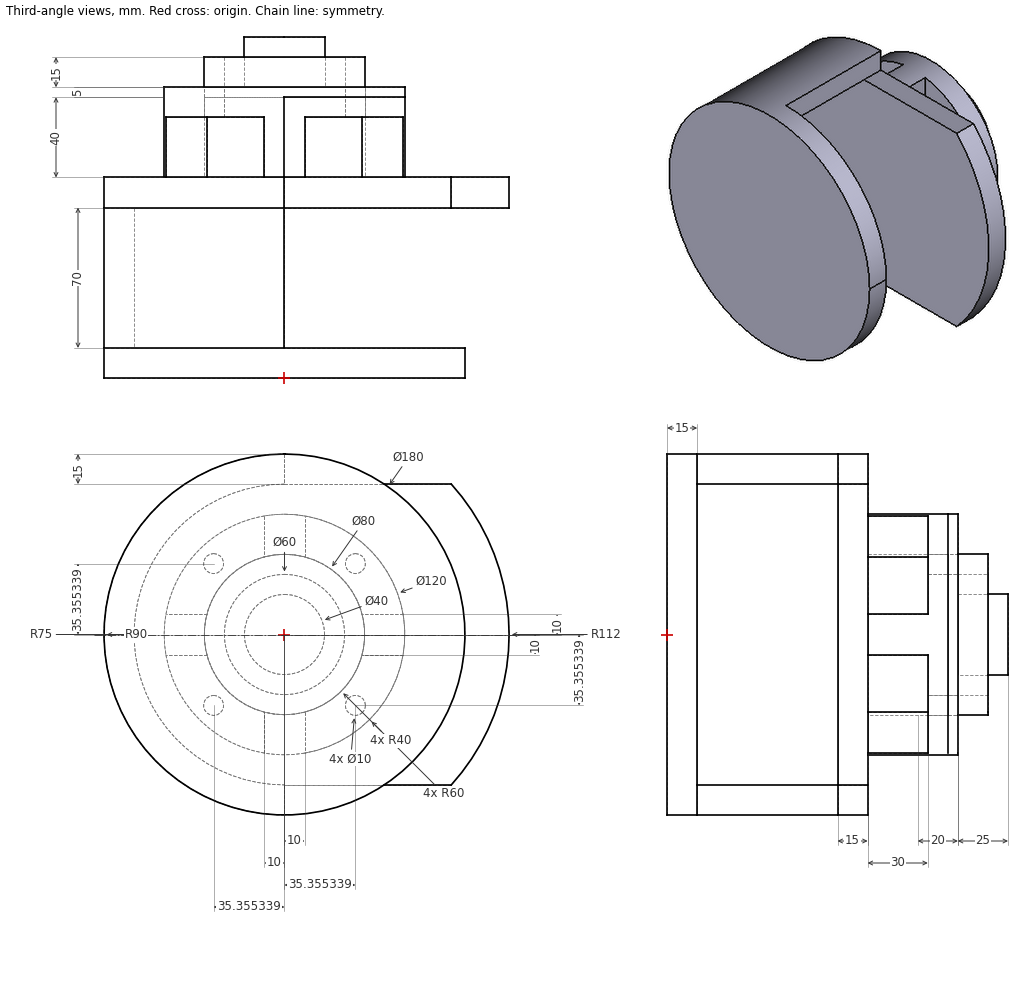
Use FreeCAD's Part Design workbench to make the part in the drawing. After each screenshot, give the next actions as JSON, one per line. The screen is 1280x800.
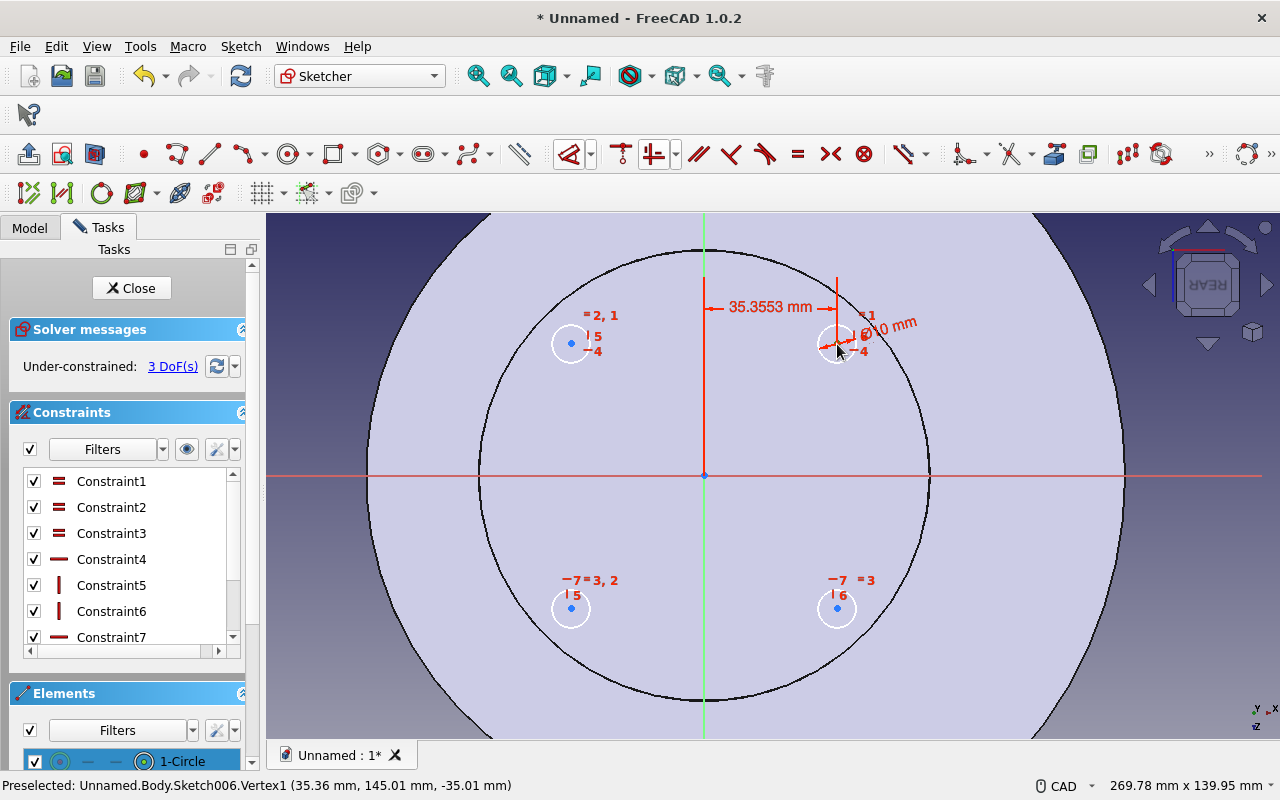
{"action": "left_click", "coordinate": [590, 154]}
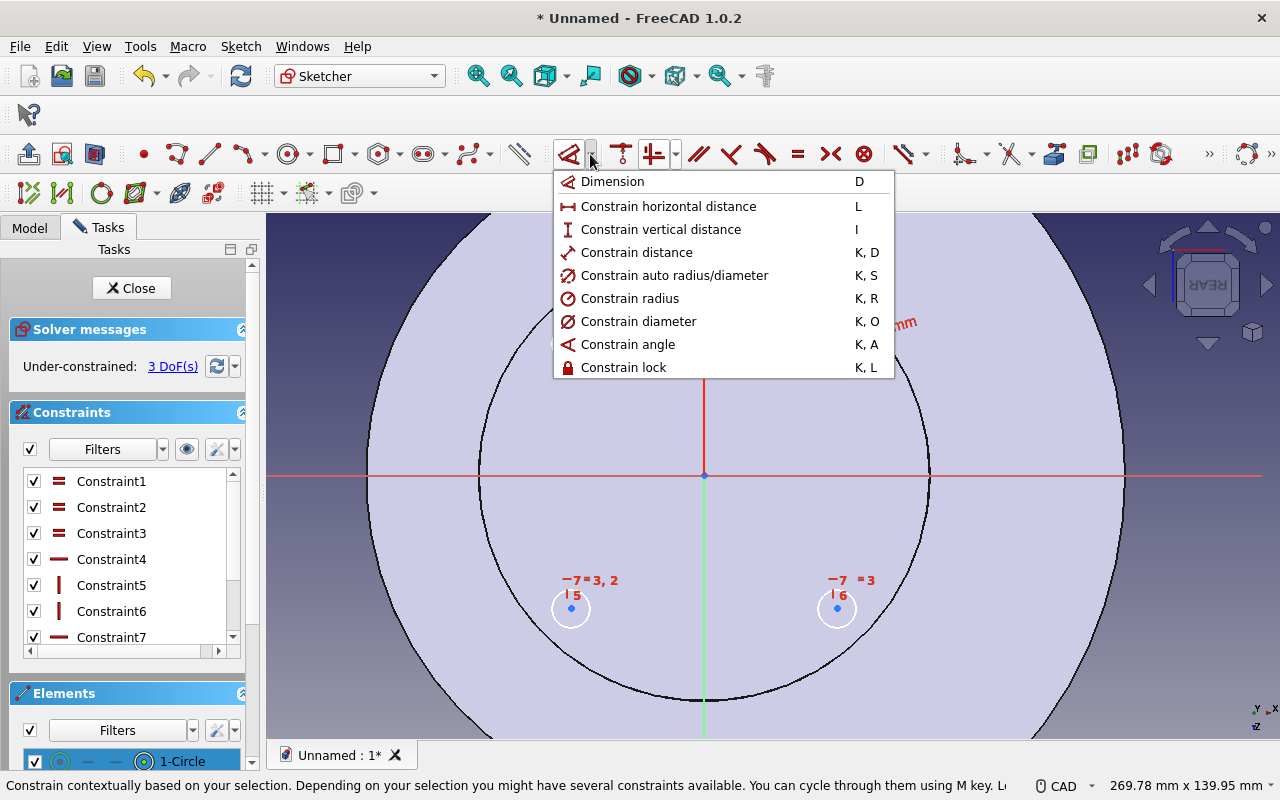
{"action": "left_click", "coordinate": [724, 230]}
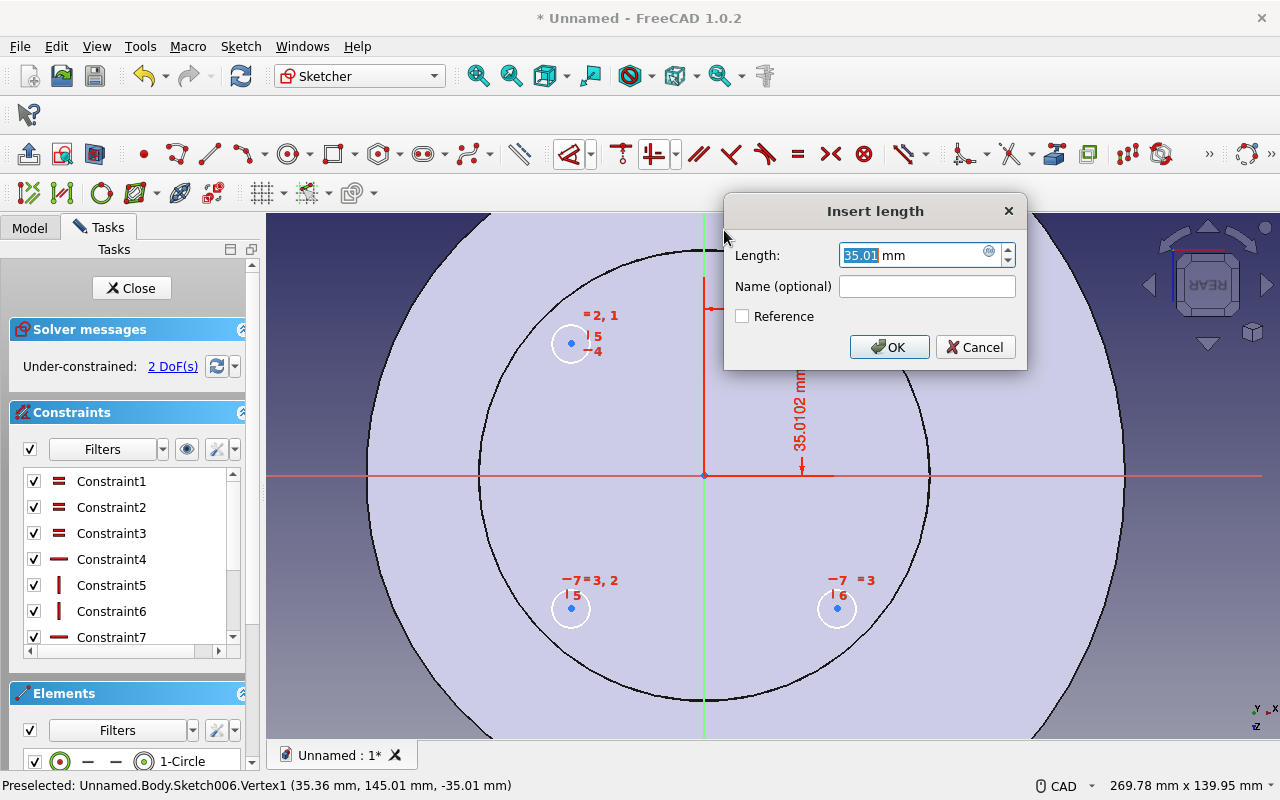
{"action": "type", "text": "35.355339"}
{"action": "key", "text": "Return"}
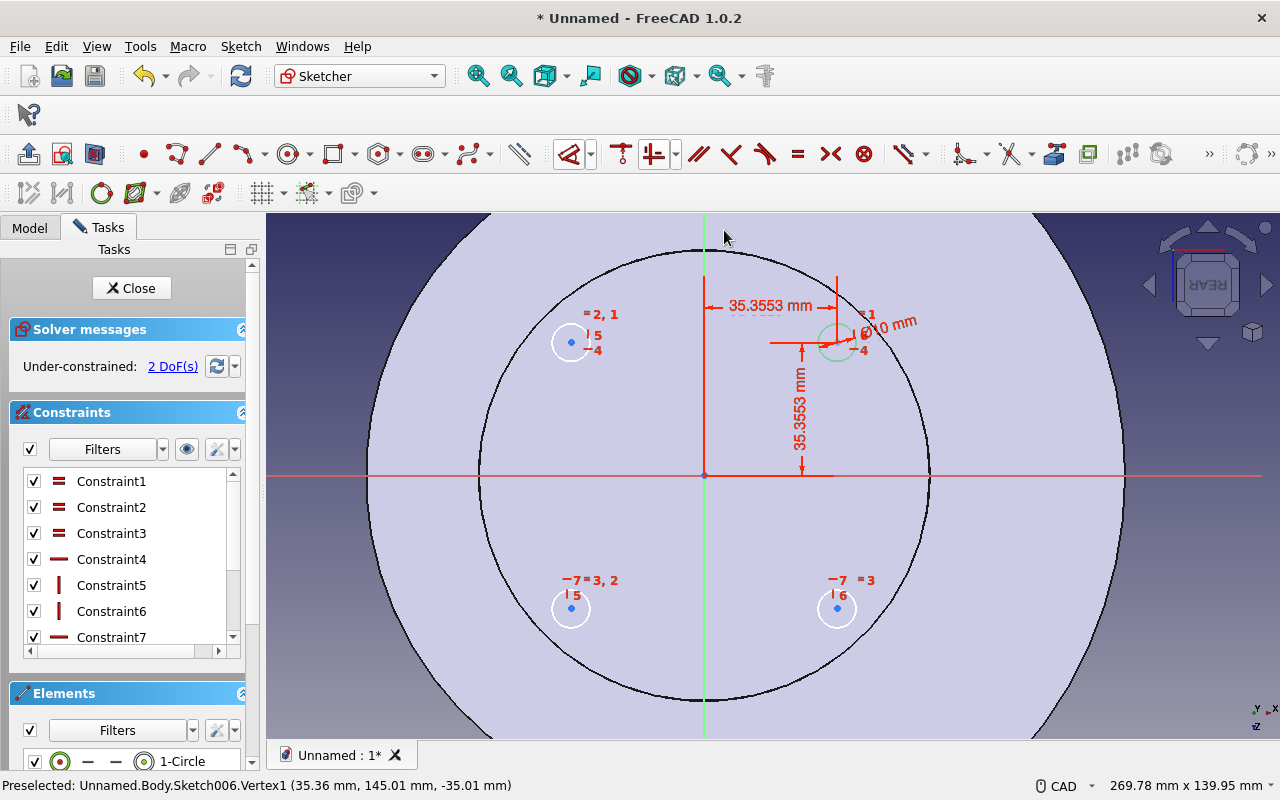
{"action": "left_click", "coordinate": [571, 343]}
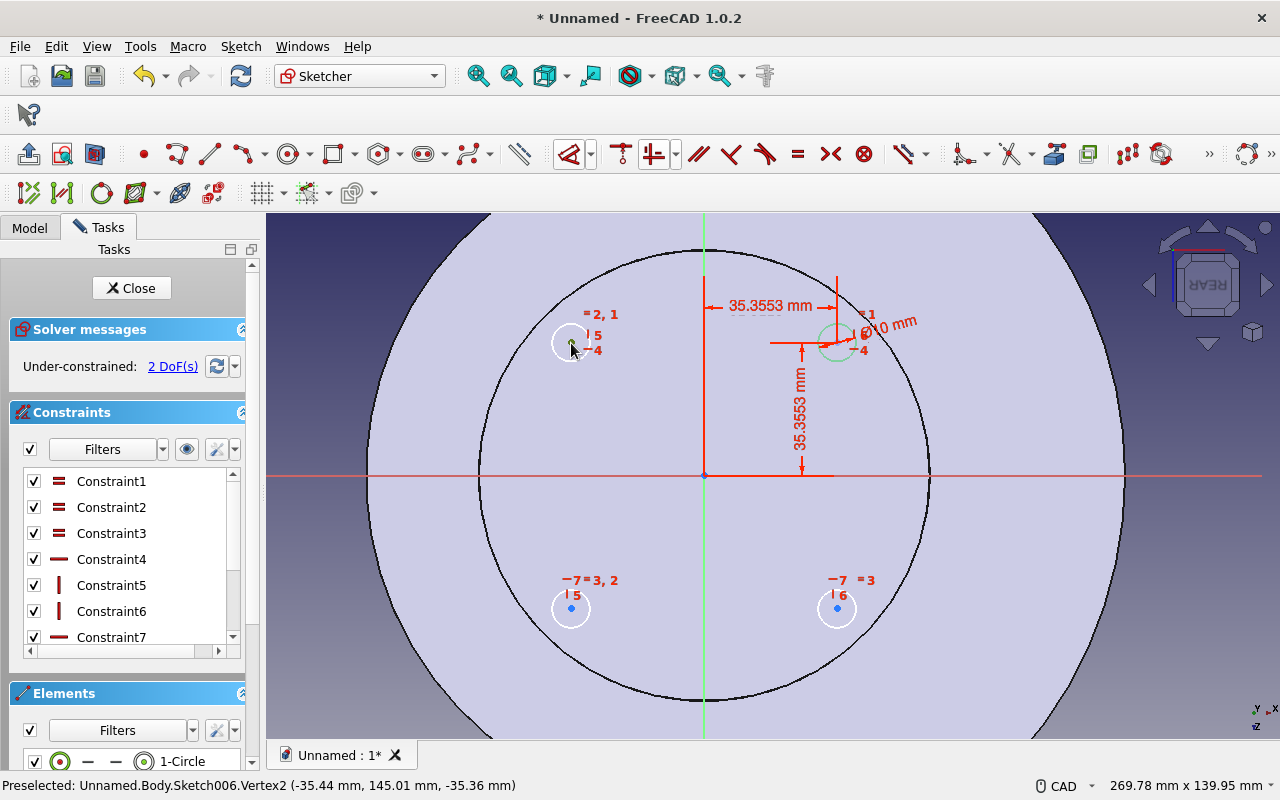
{"action": "key", "text": "l"}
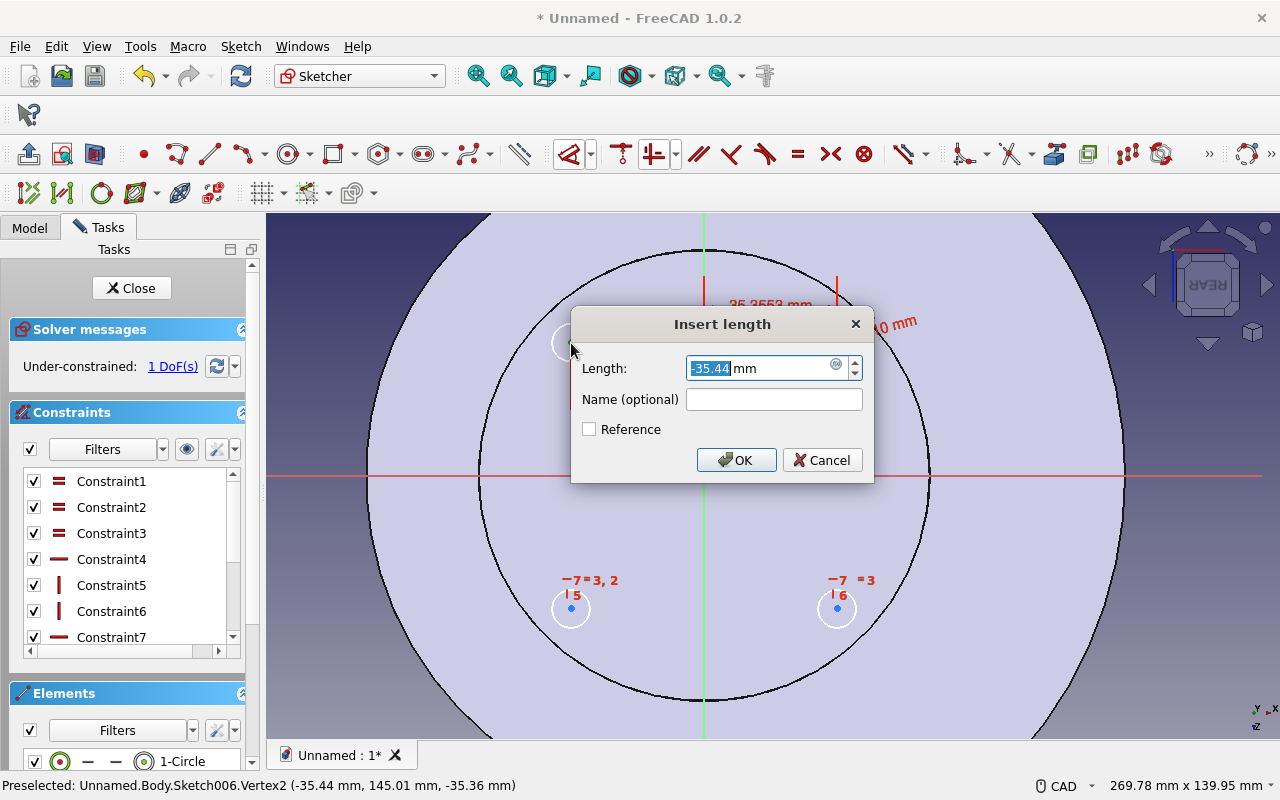
{"action": "type", "text": "-35.355339"}
{"action": "key", "text": "Return"}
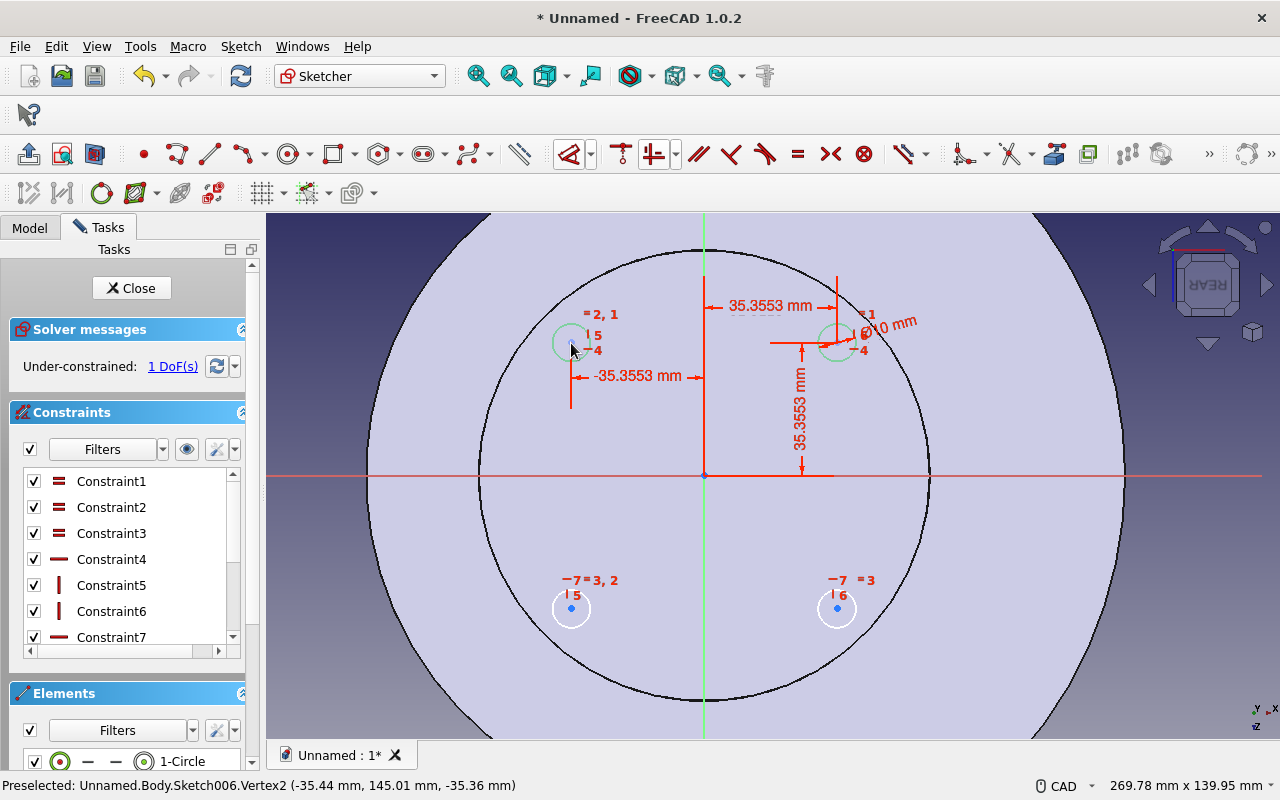
{"action": "left_click", "coordinate": [571, 609]}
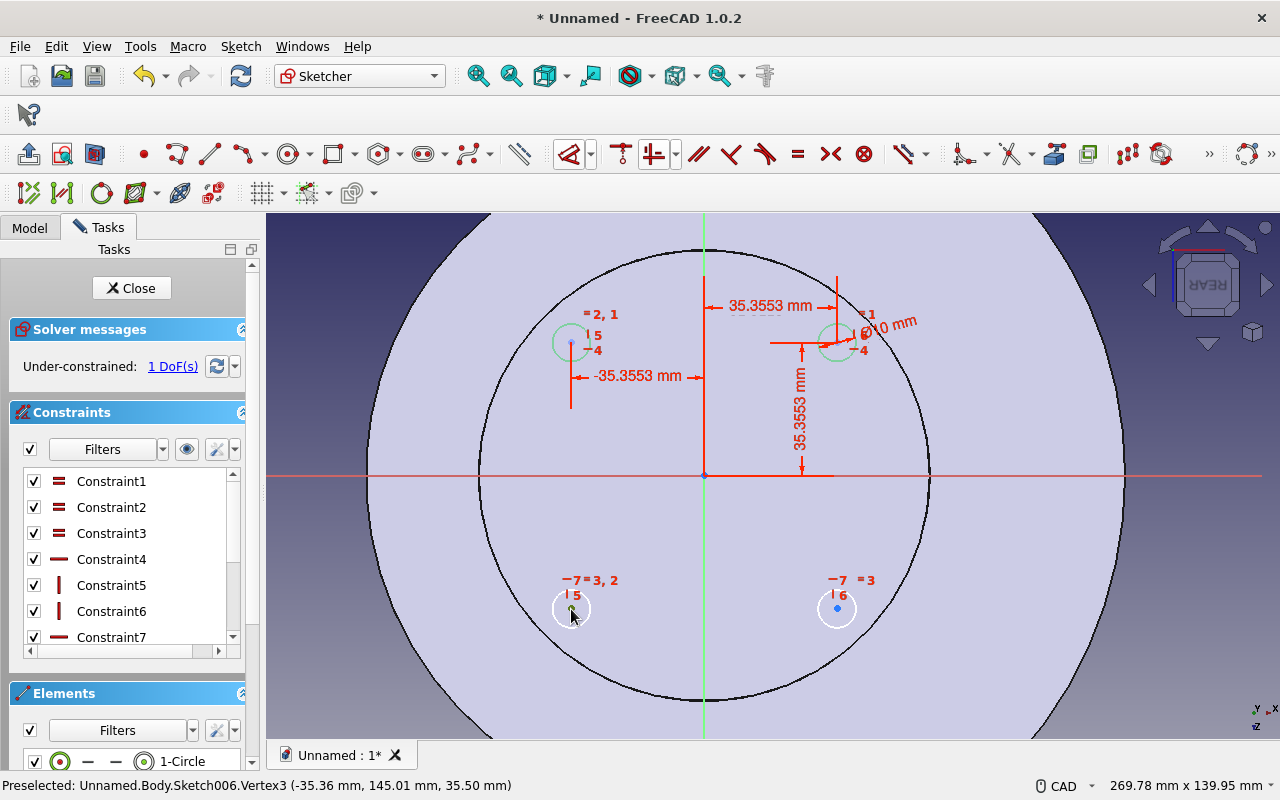
{"action": "key", "text": "i"}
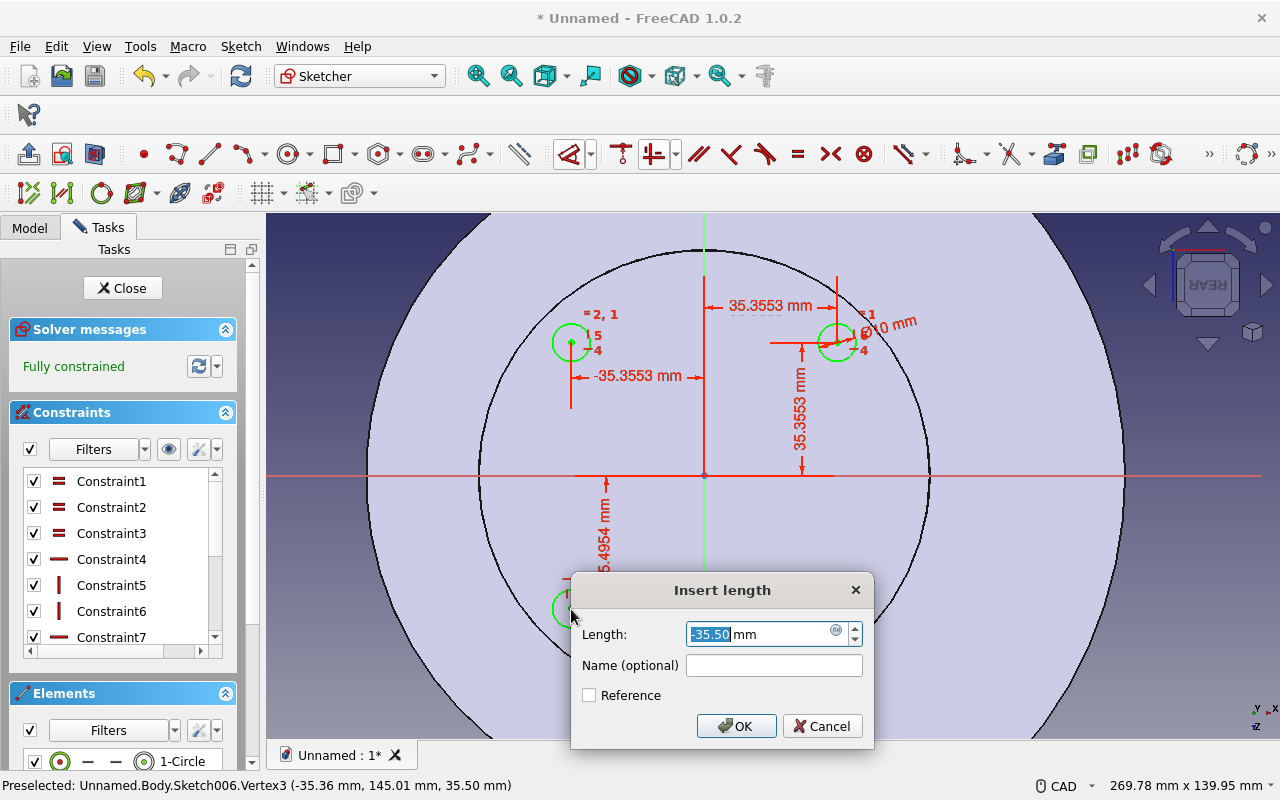
{"action": "type", "text": "-35.355339"}
{"action": "key", "text": "Return"}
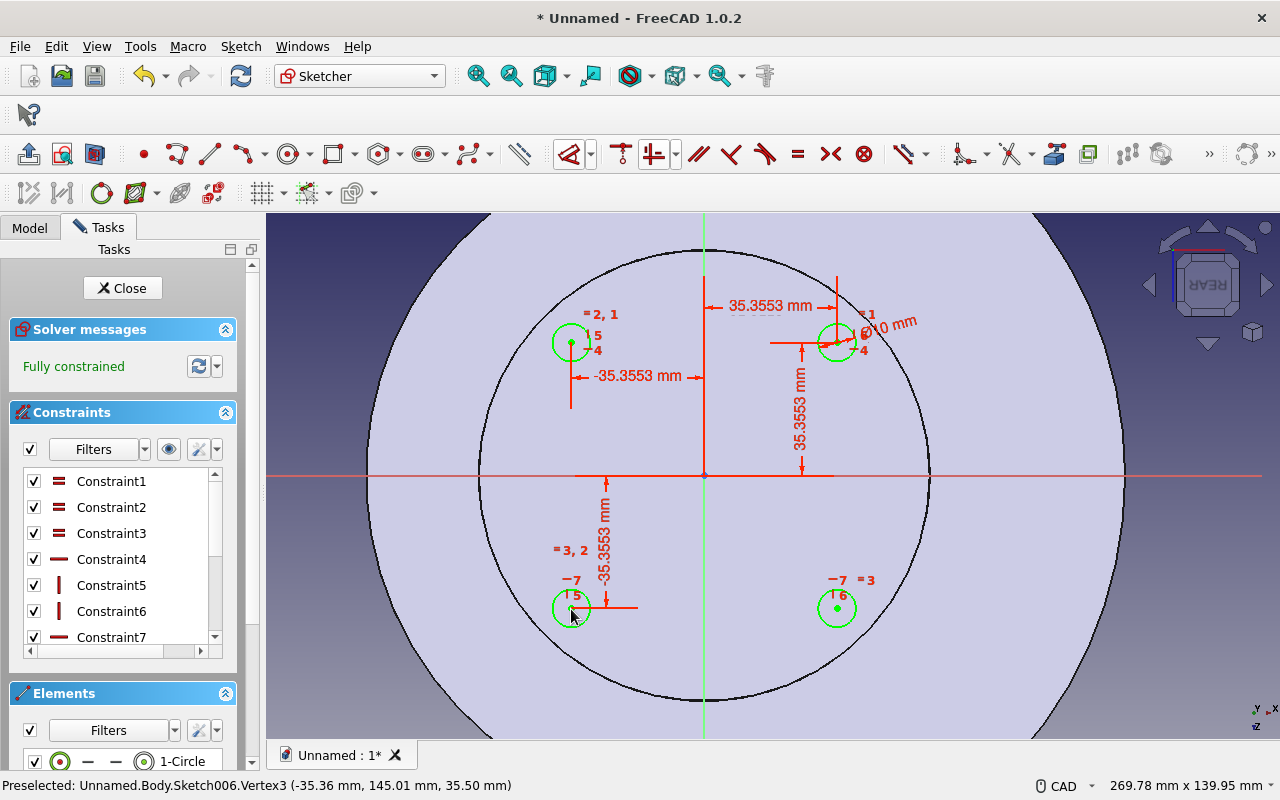
{"action": "left_click", "coordinate": [123, 288]}